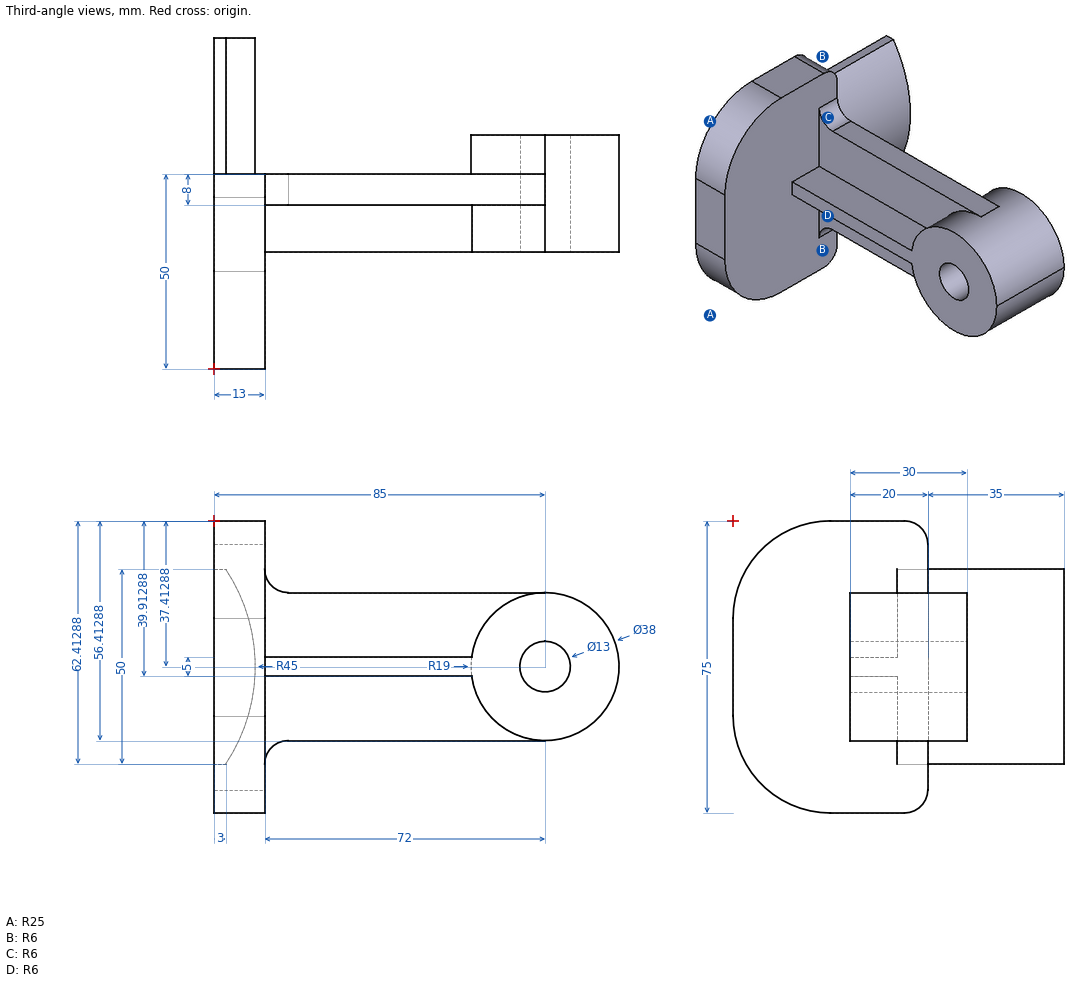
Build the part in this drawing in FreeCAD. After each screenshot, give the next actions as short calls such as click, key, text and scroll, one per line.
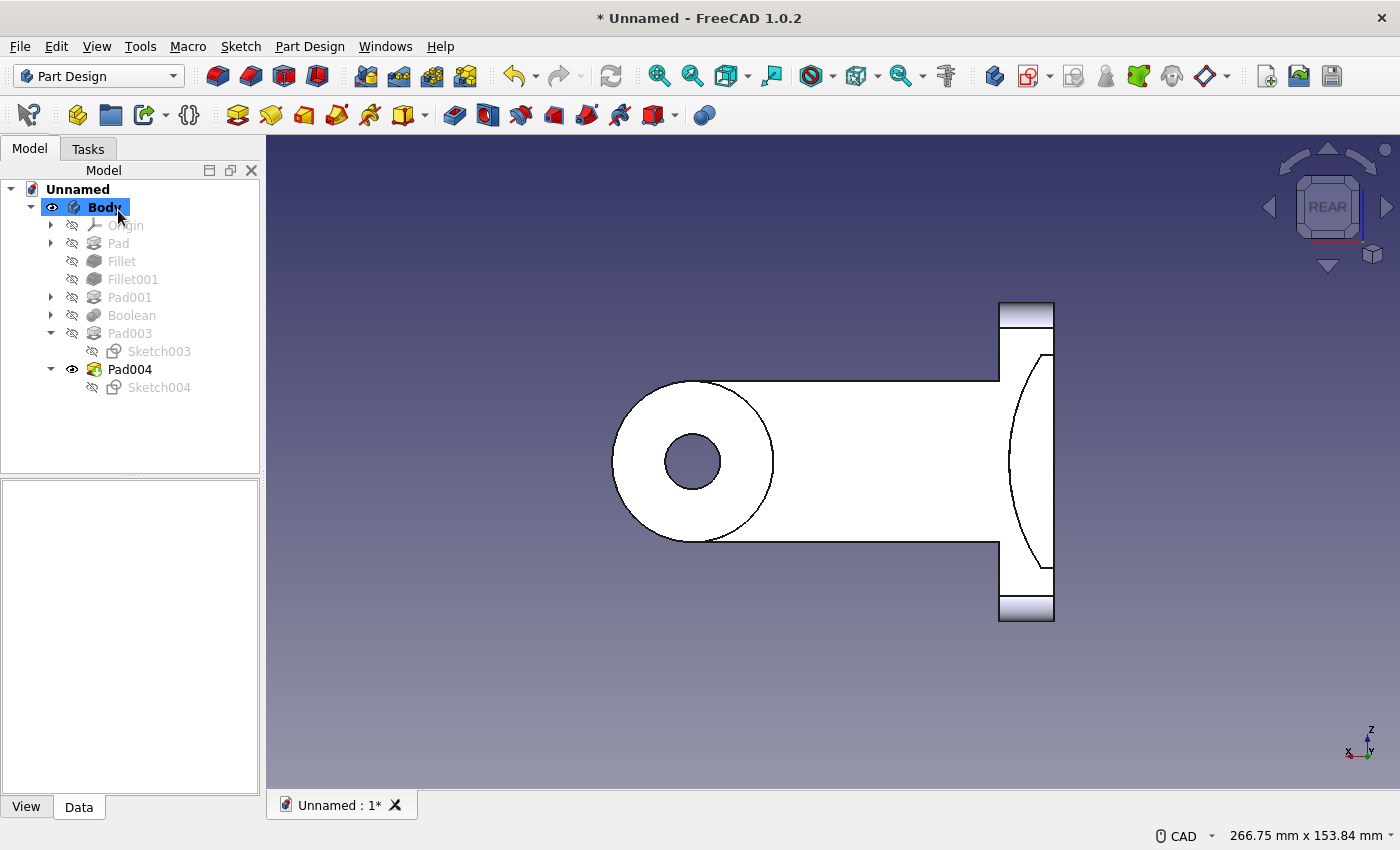
key(6)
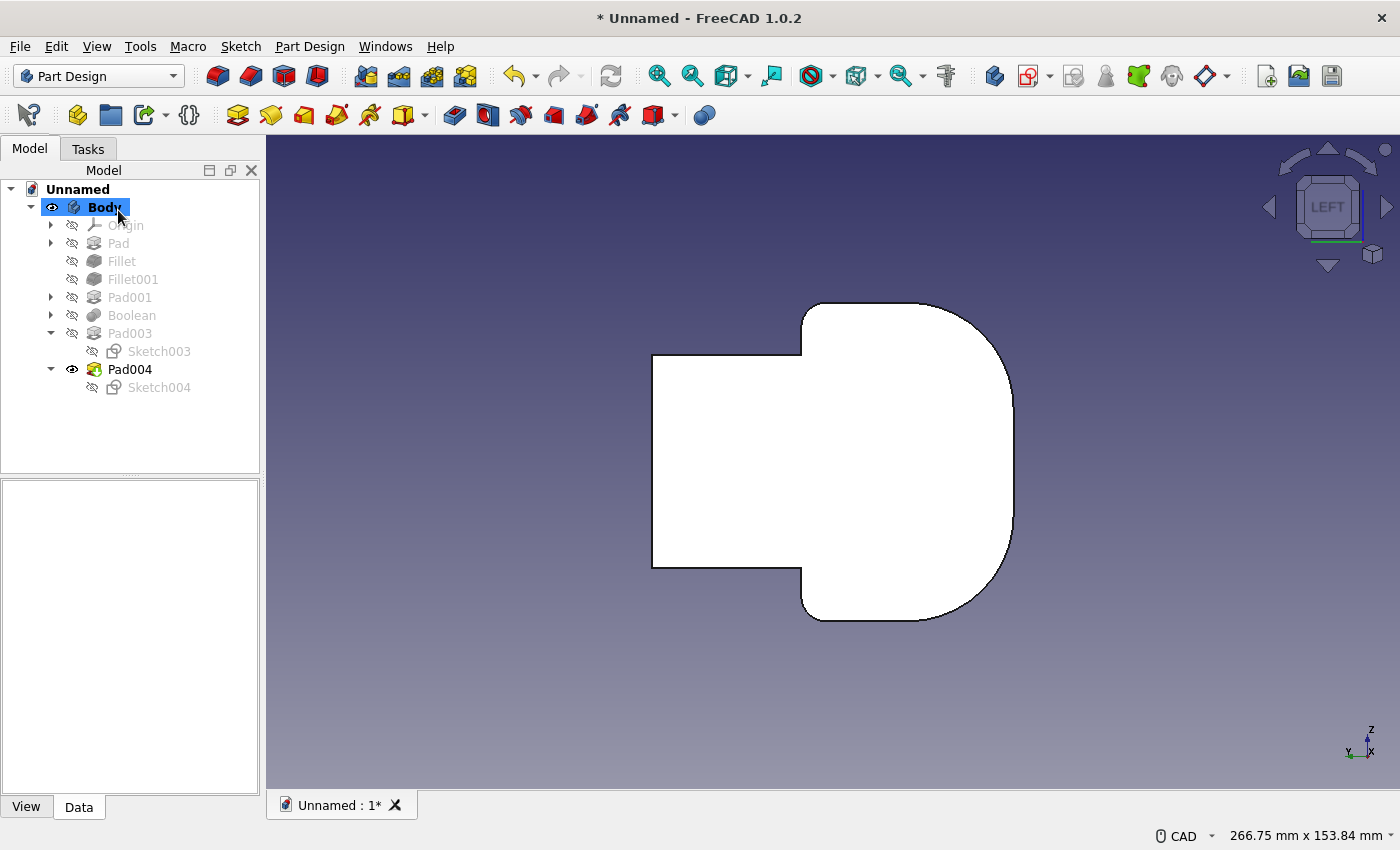
key(v)
key(3)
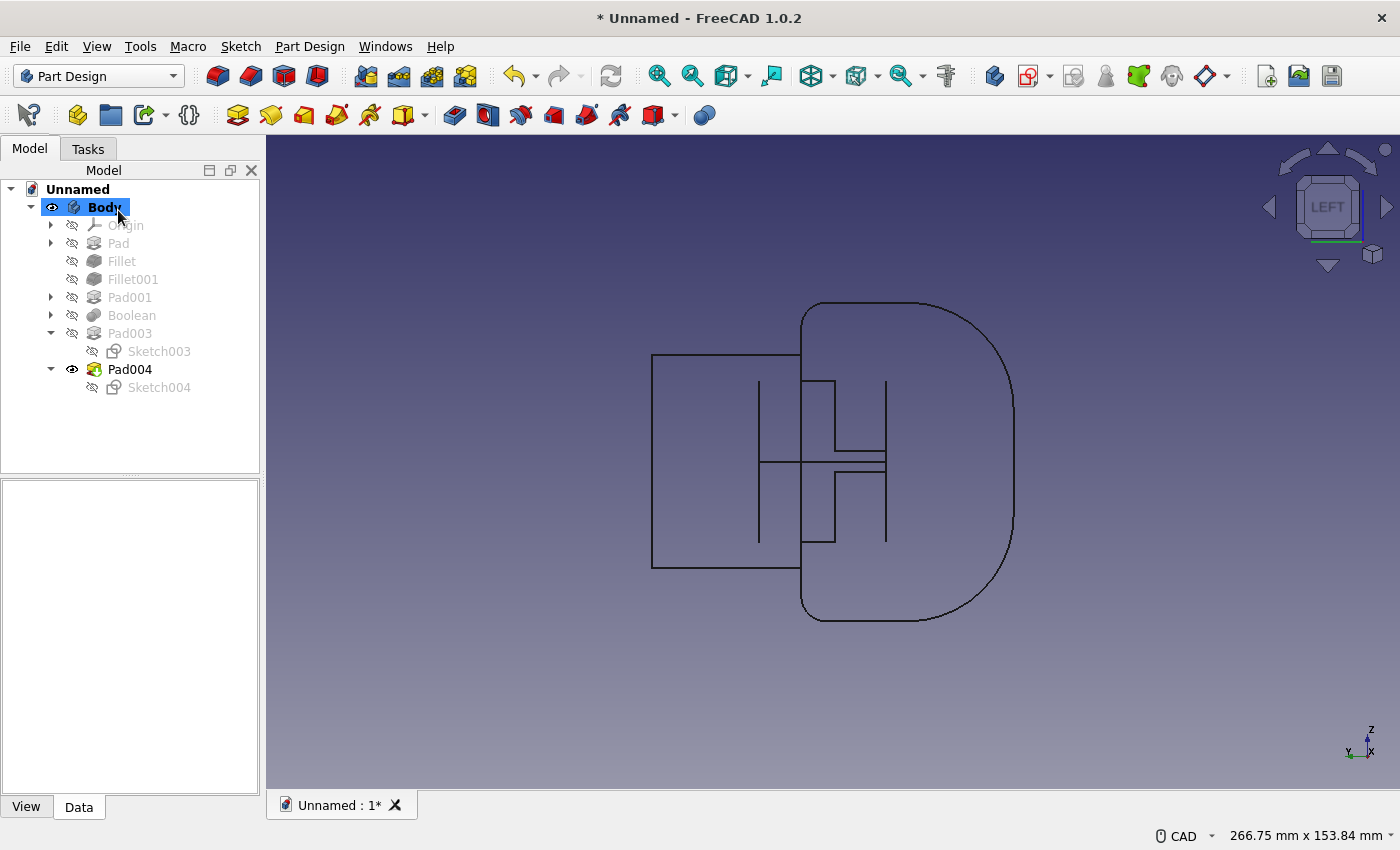
key(0)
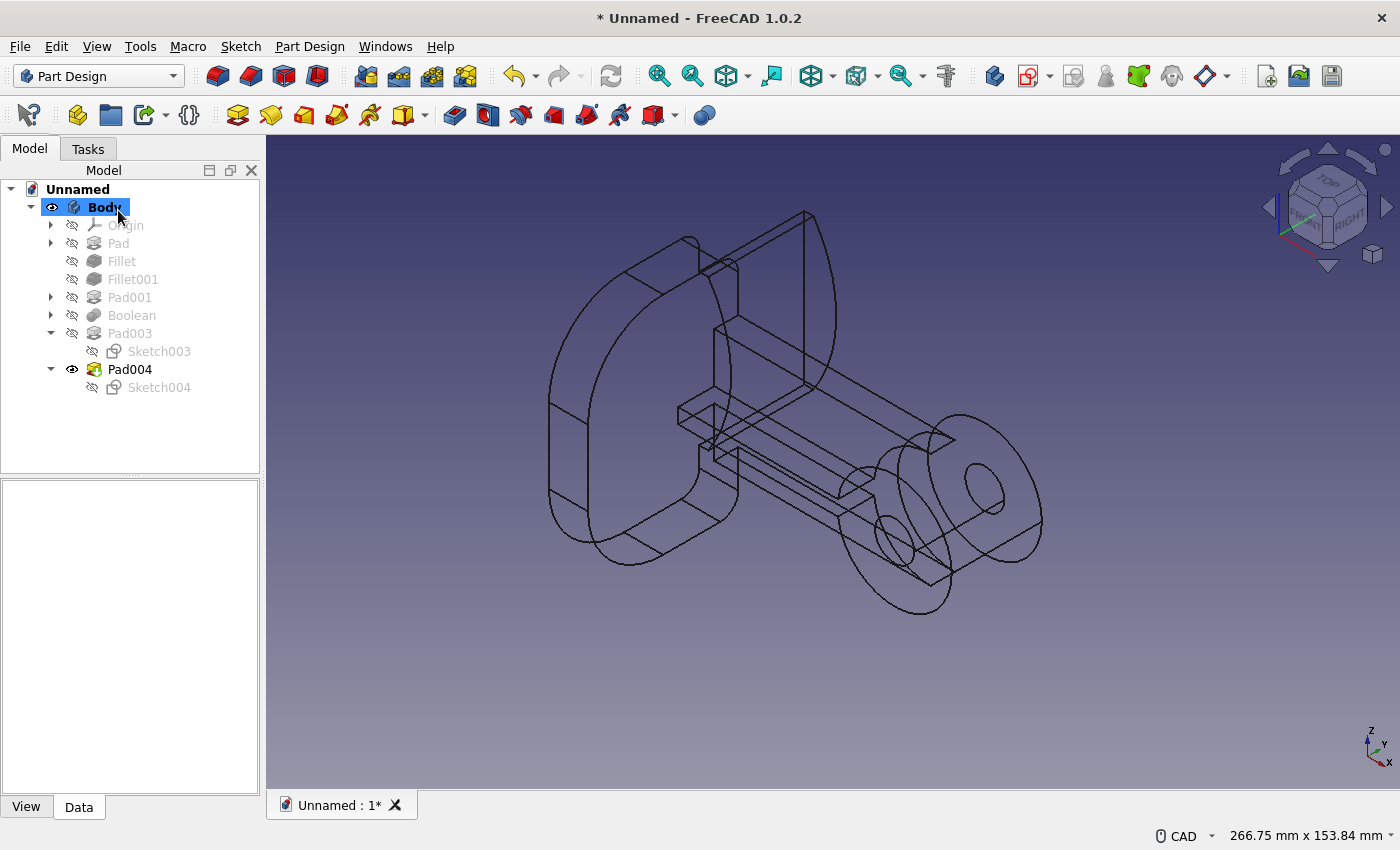
click(726, 321)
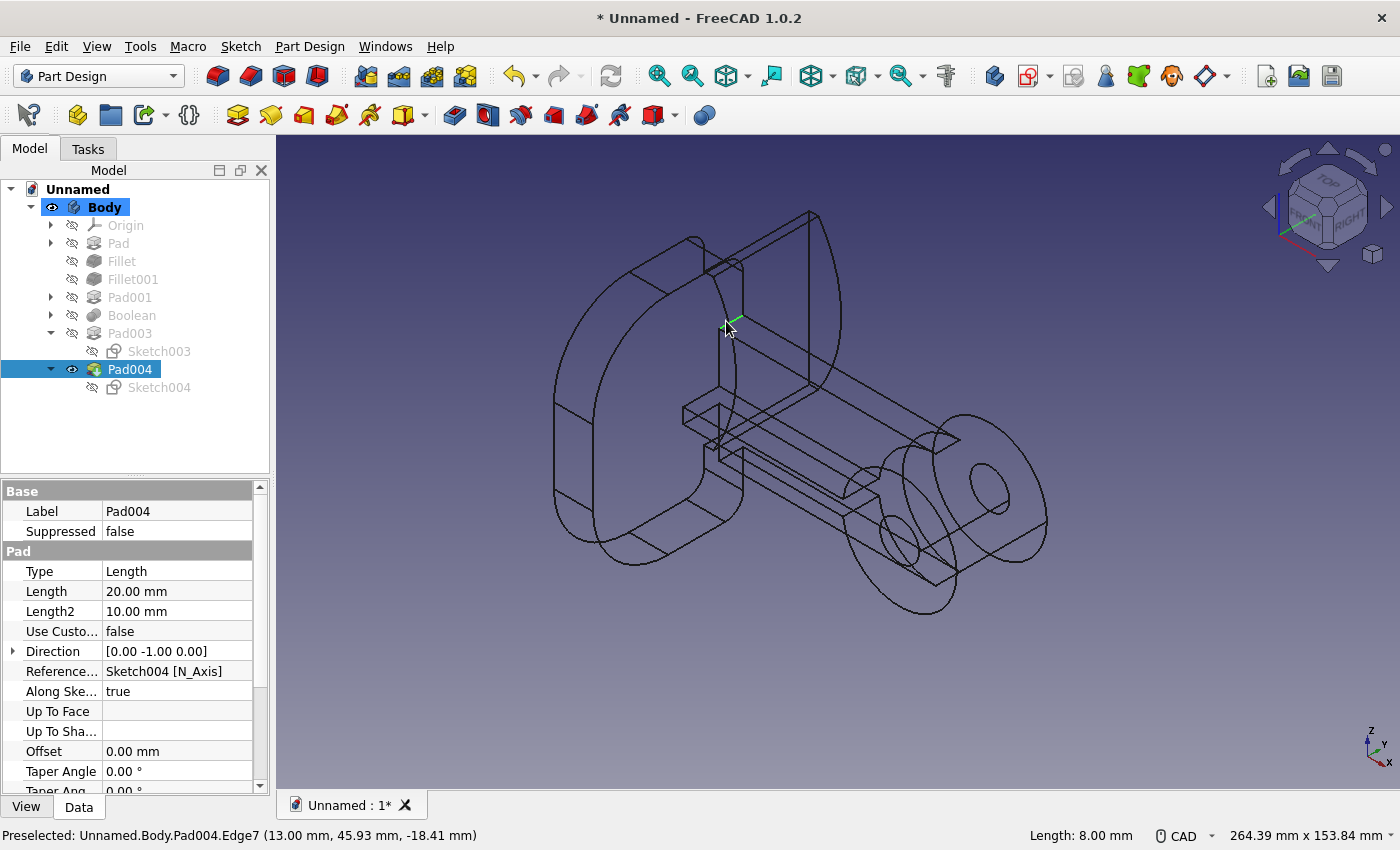
key(v)
key(1)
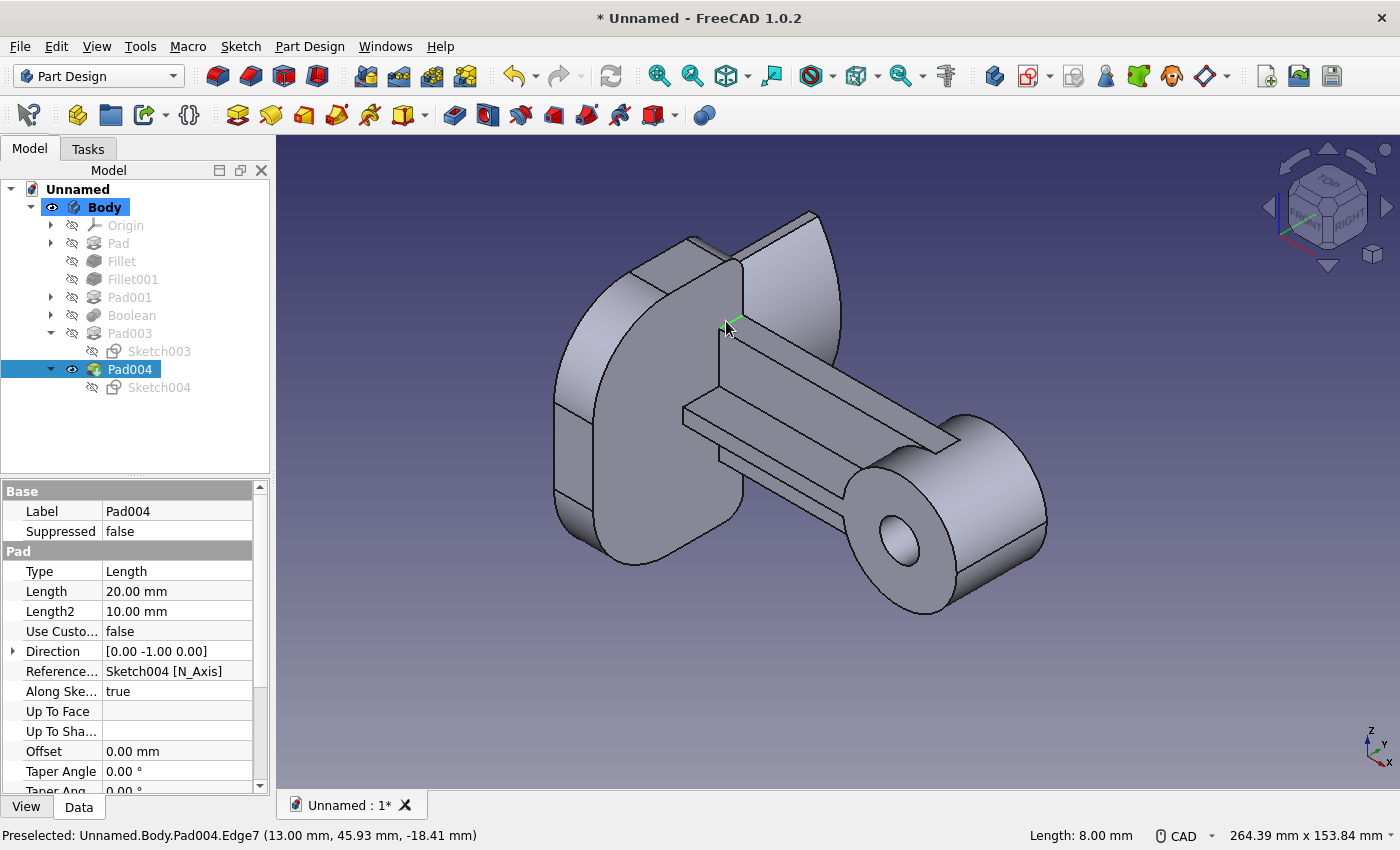
click(218, 76)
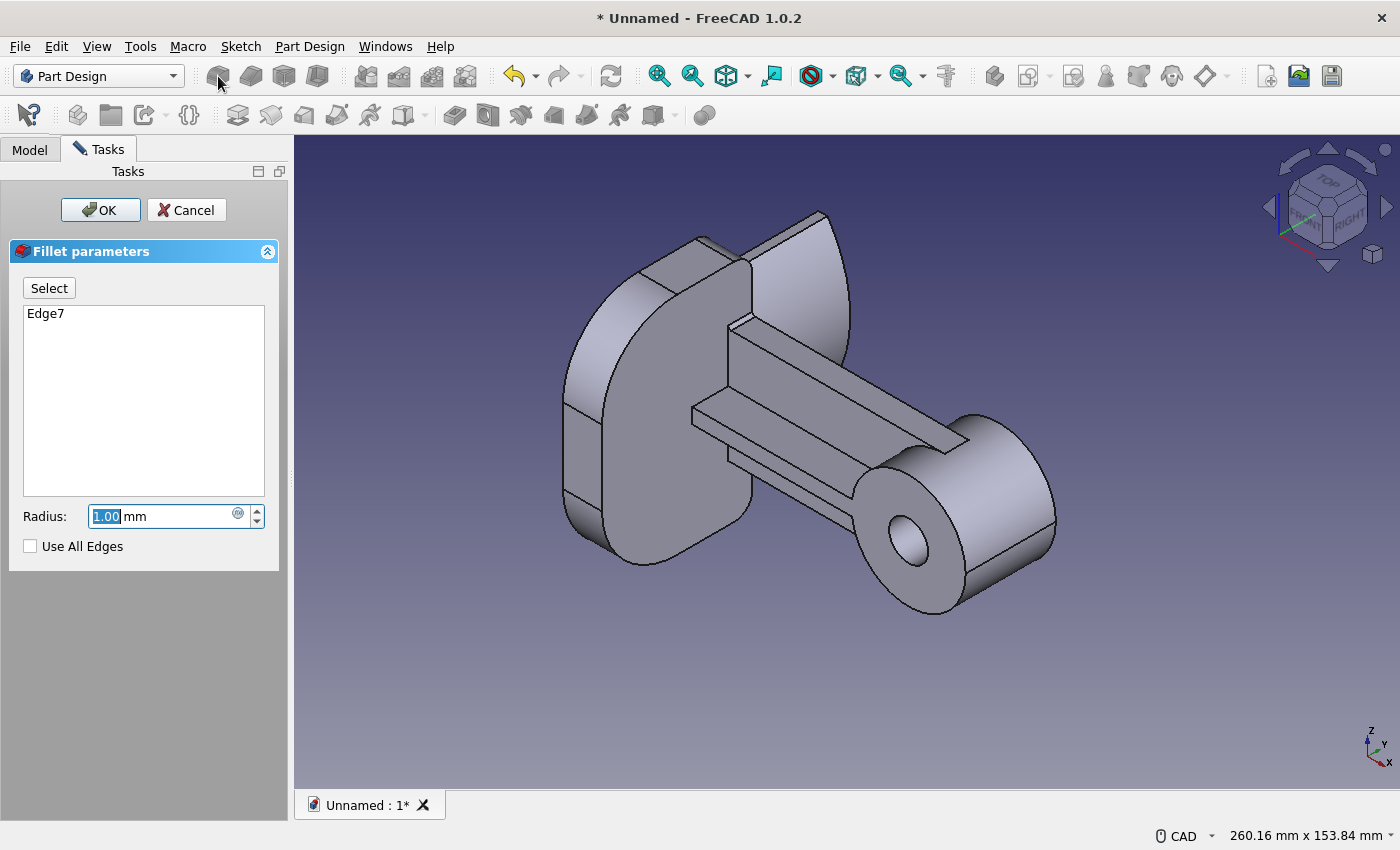
text(6)
key(Tab)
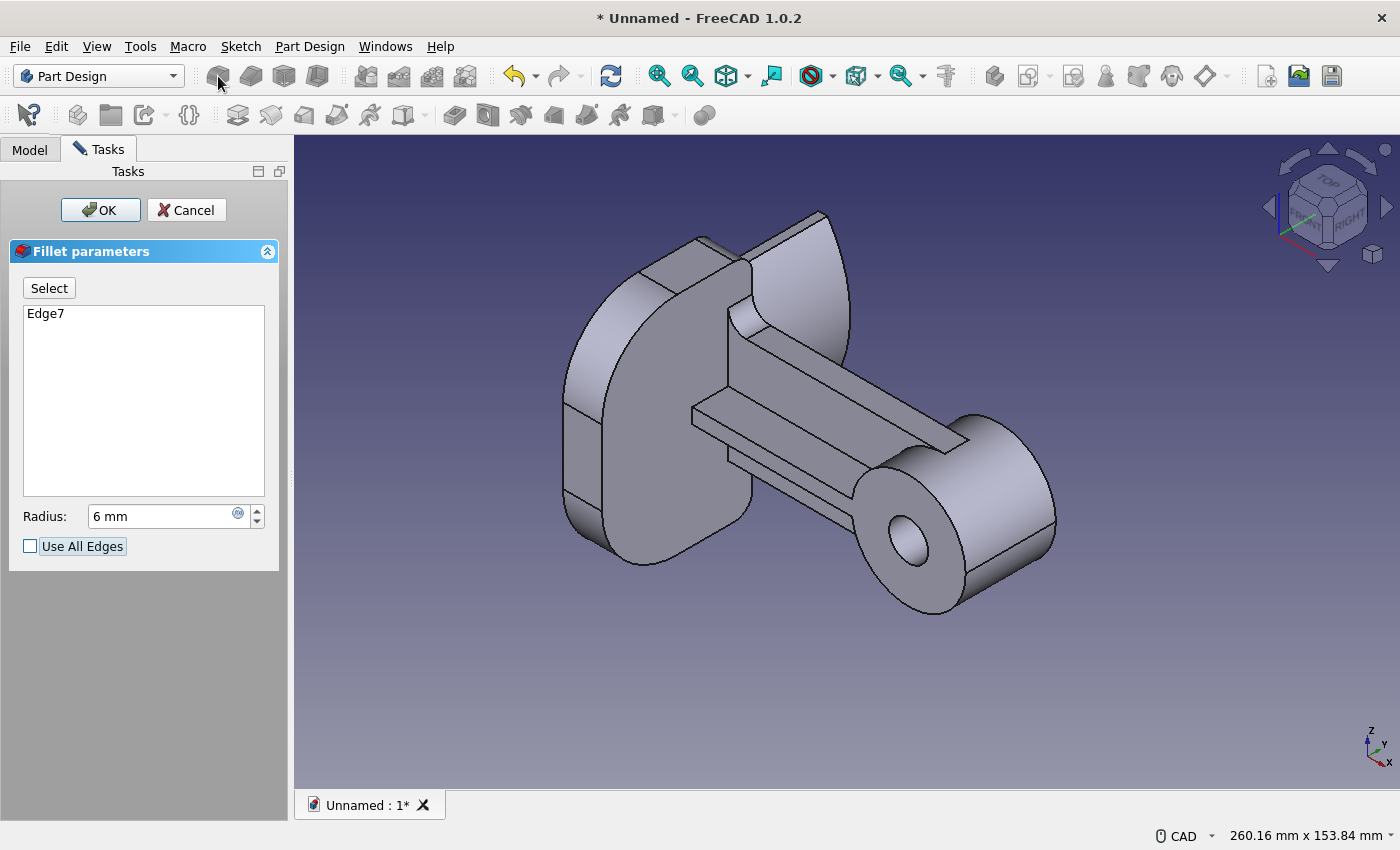
click(101, 210)